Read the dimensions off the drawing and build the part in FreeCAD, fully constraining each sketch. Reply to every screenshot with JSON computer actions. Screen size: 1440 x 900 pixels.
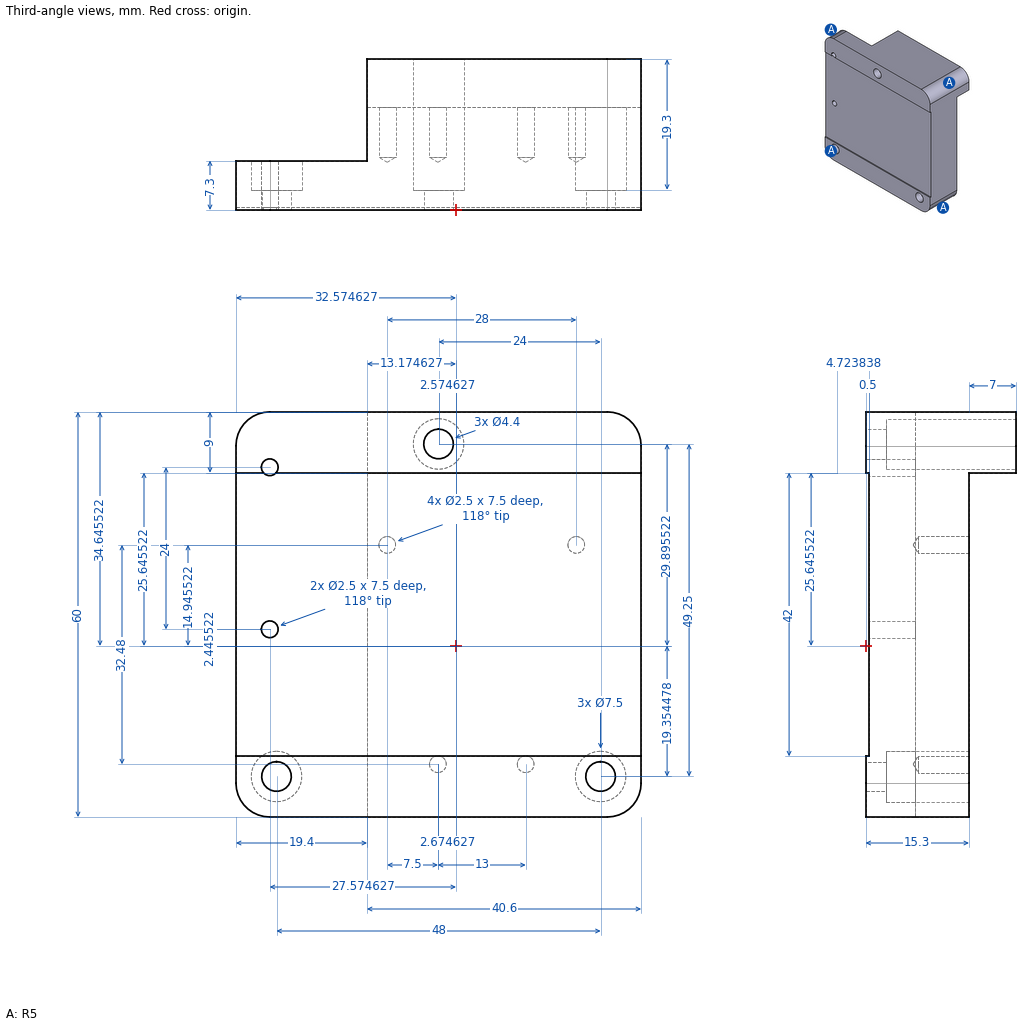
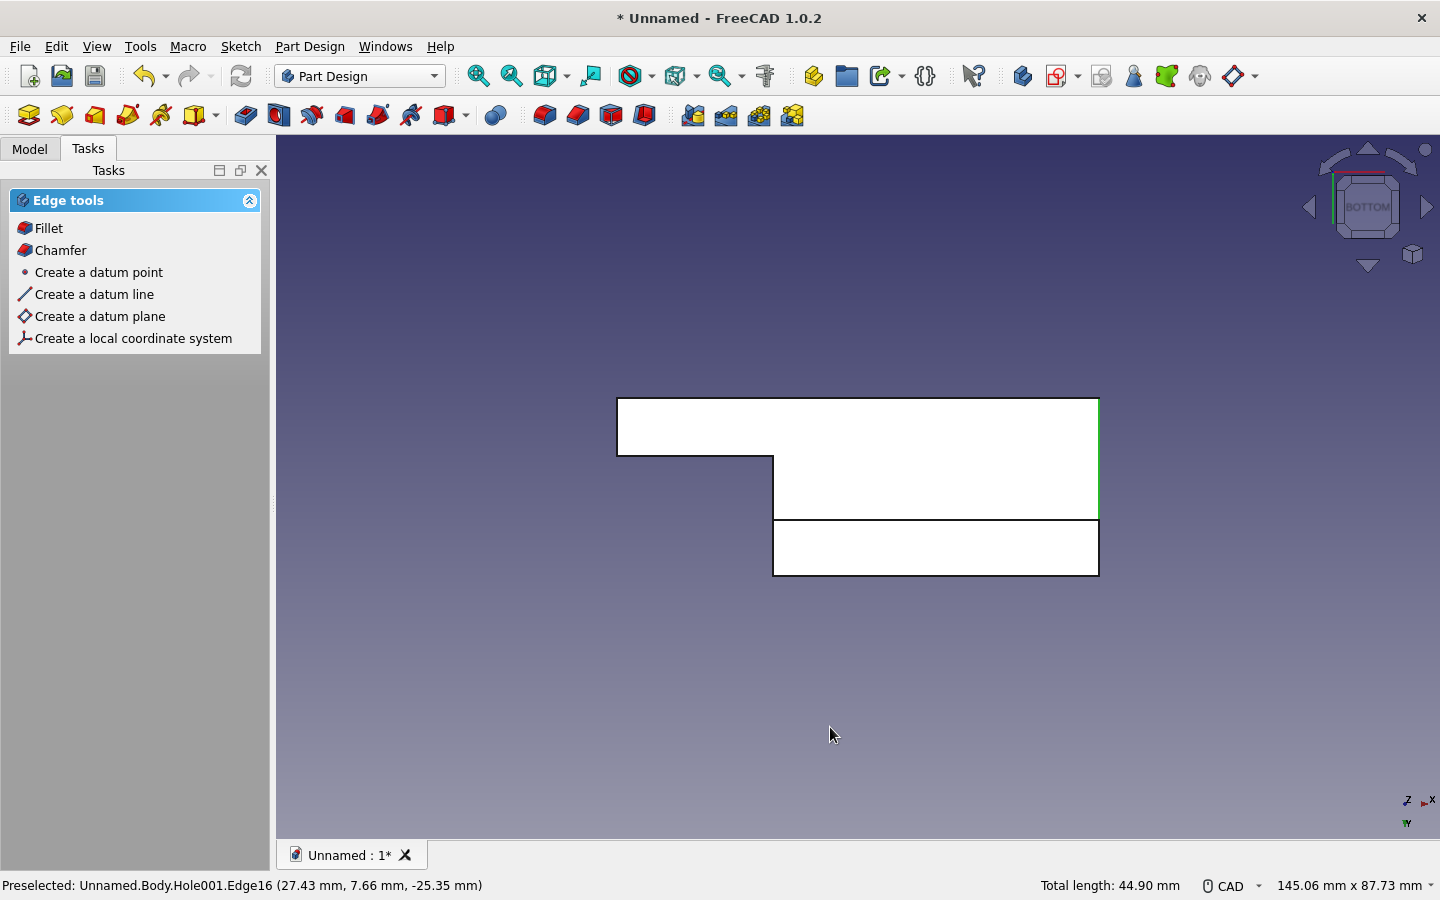
{"action": "key", "text": "v f"}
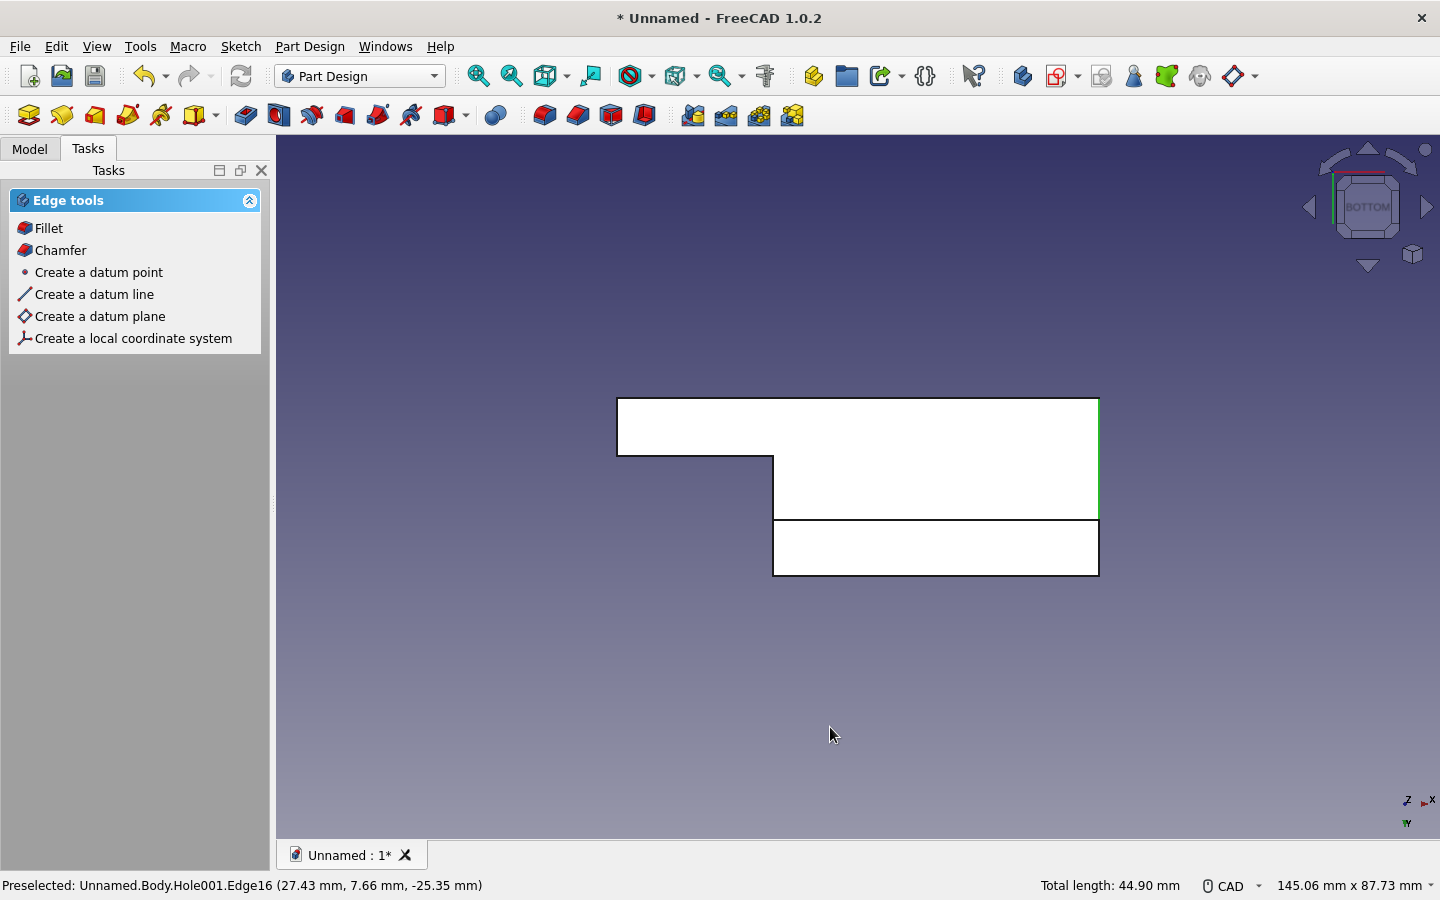
{"action": "left_click", "coordinate": [617, 426], "text": "ctrl"}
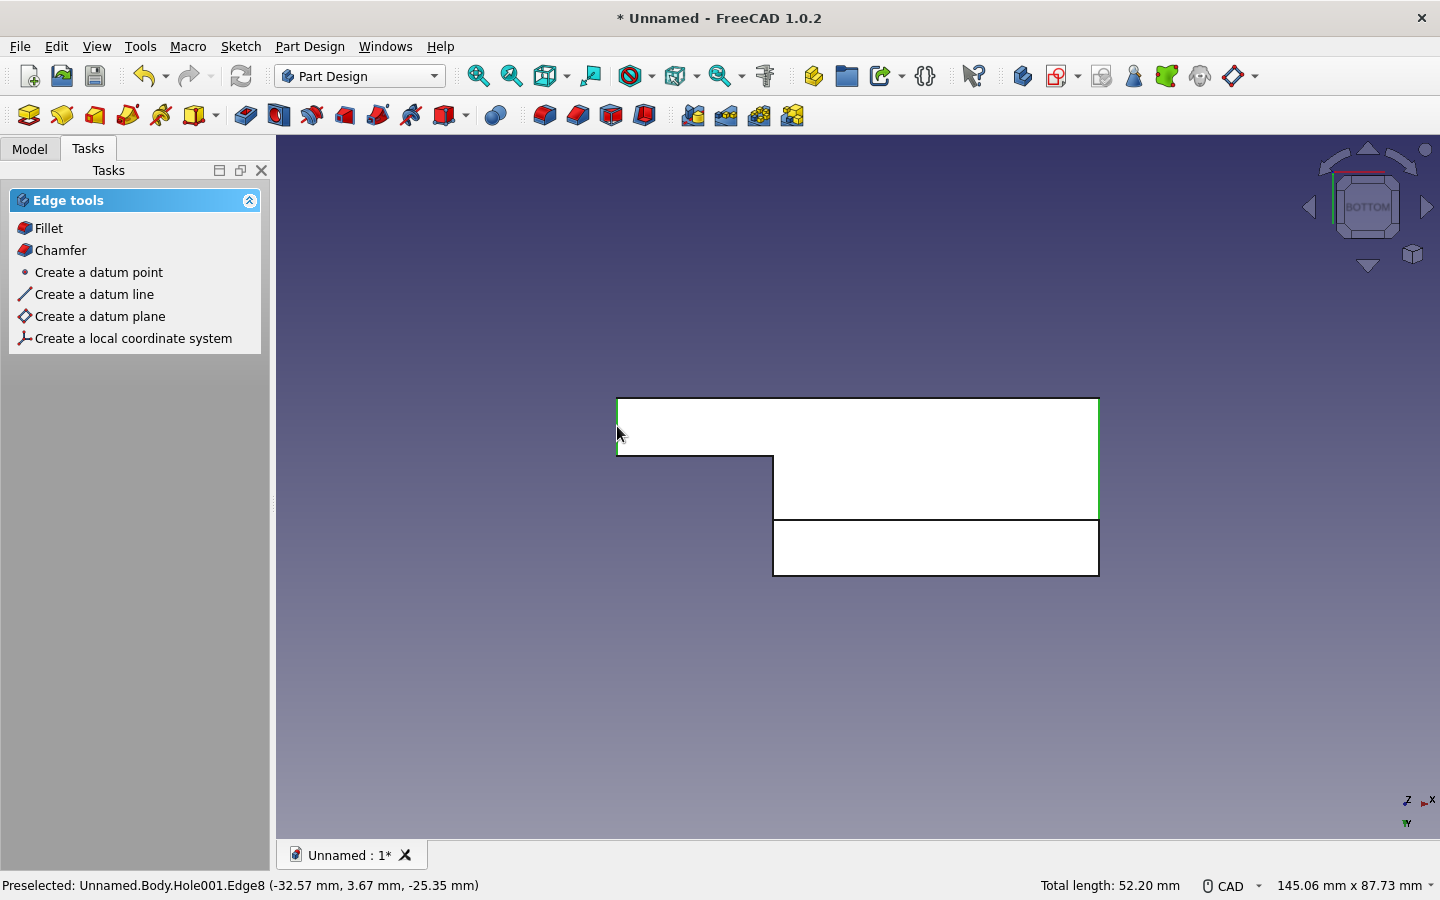
{"action": "left_click", "coordinate": [545, 116]}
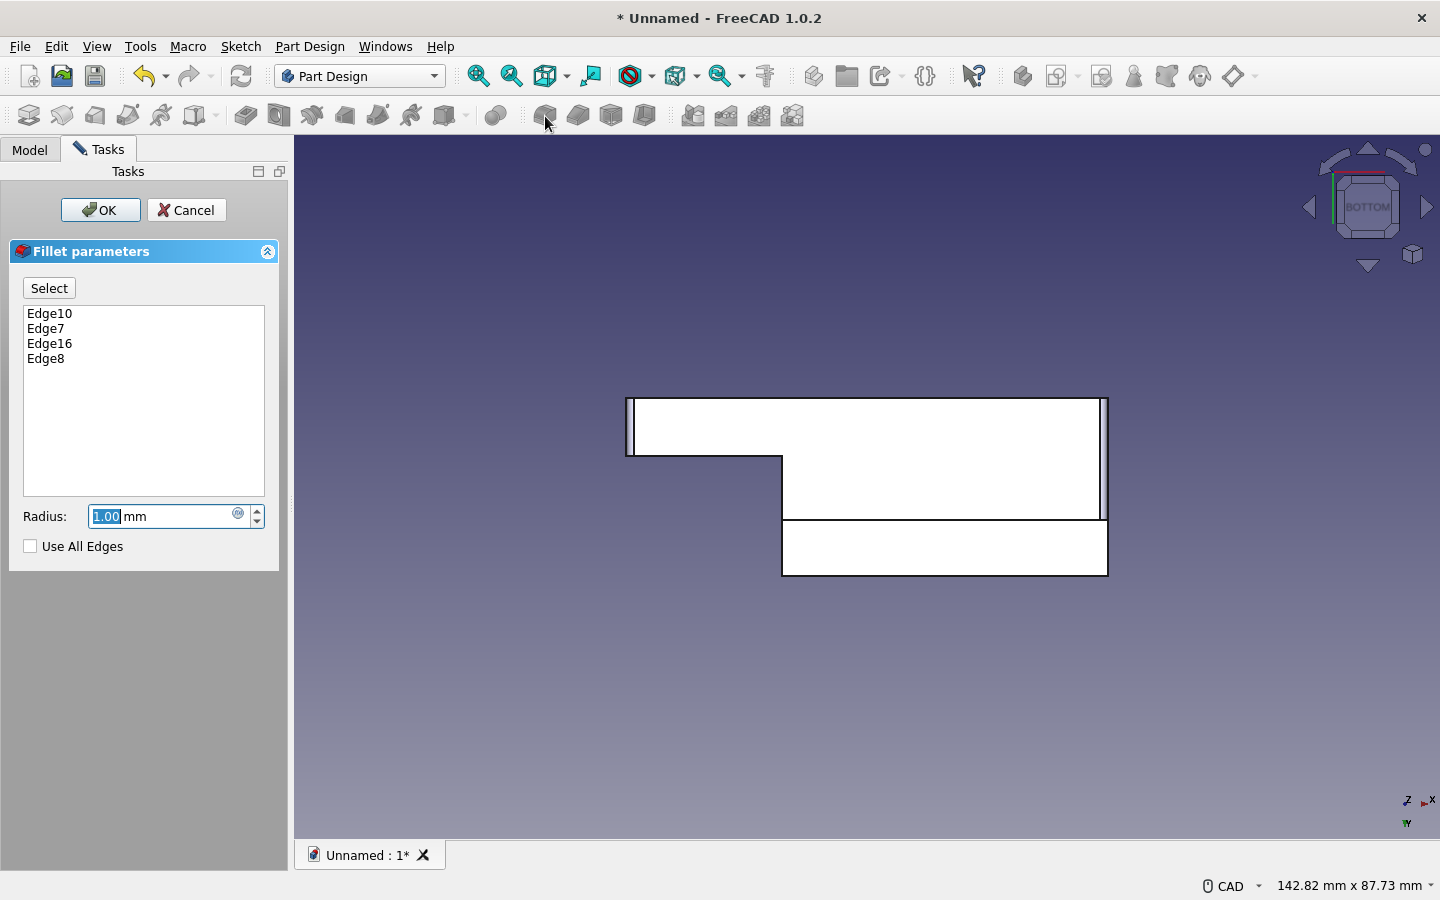
{"action": "type", "text": "5"}
{"action": "key", "text": "Tab"}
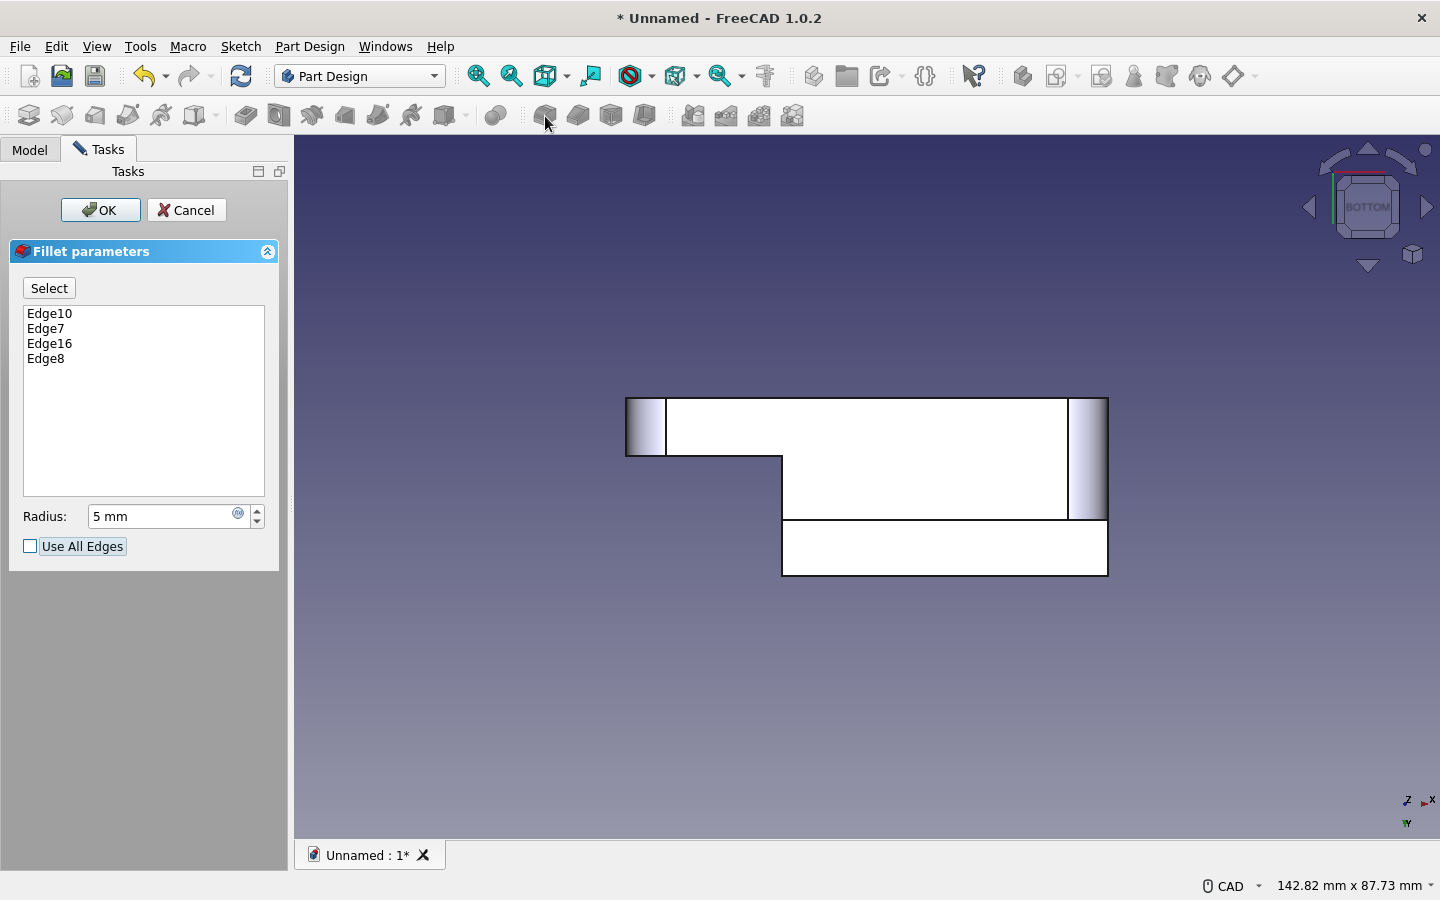
{"action": "left_click", "coordinate": [101, 210]}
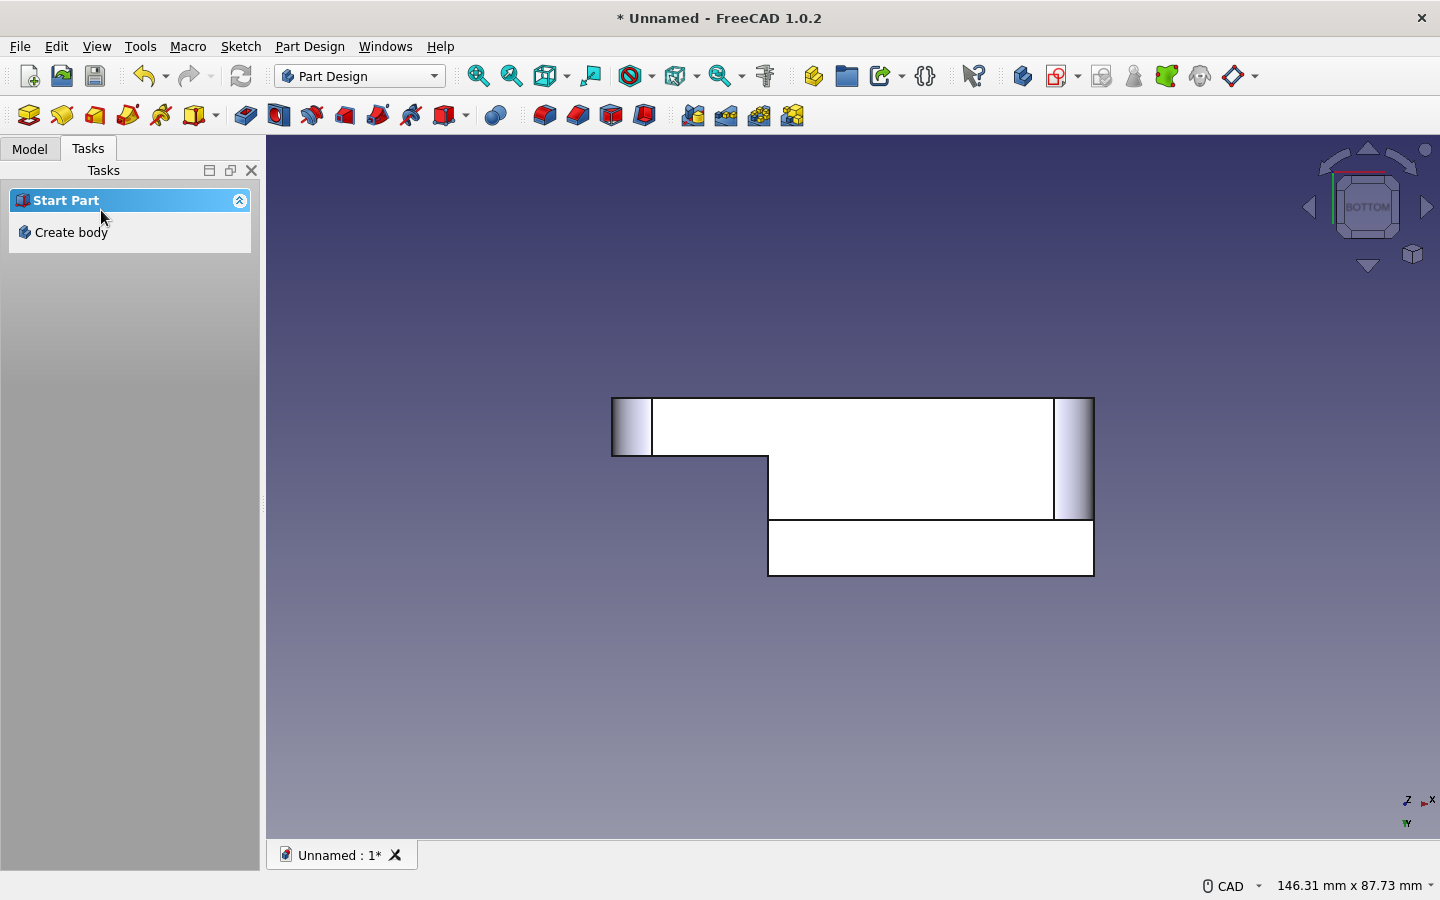
{"action": "left_click", "coordinate": [479, 76]}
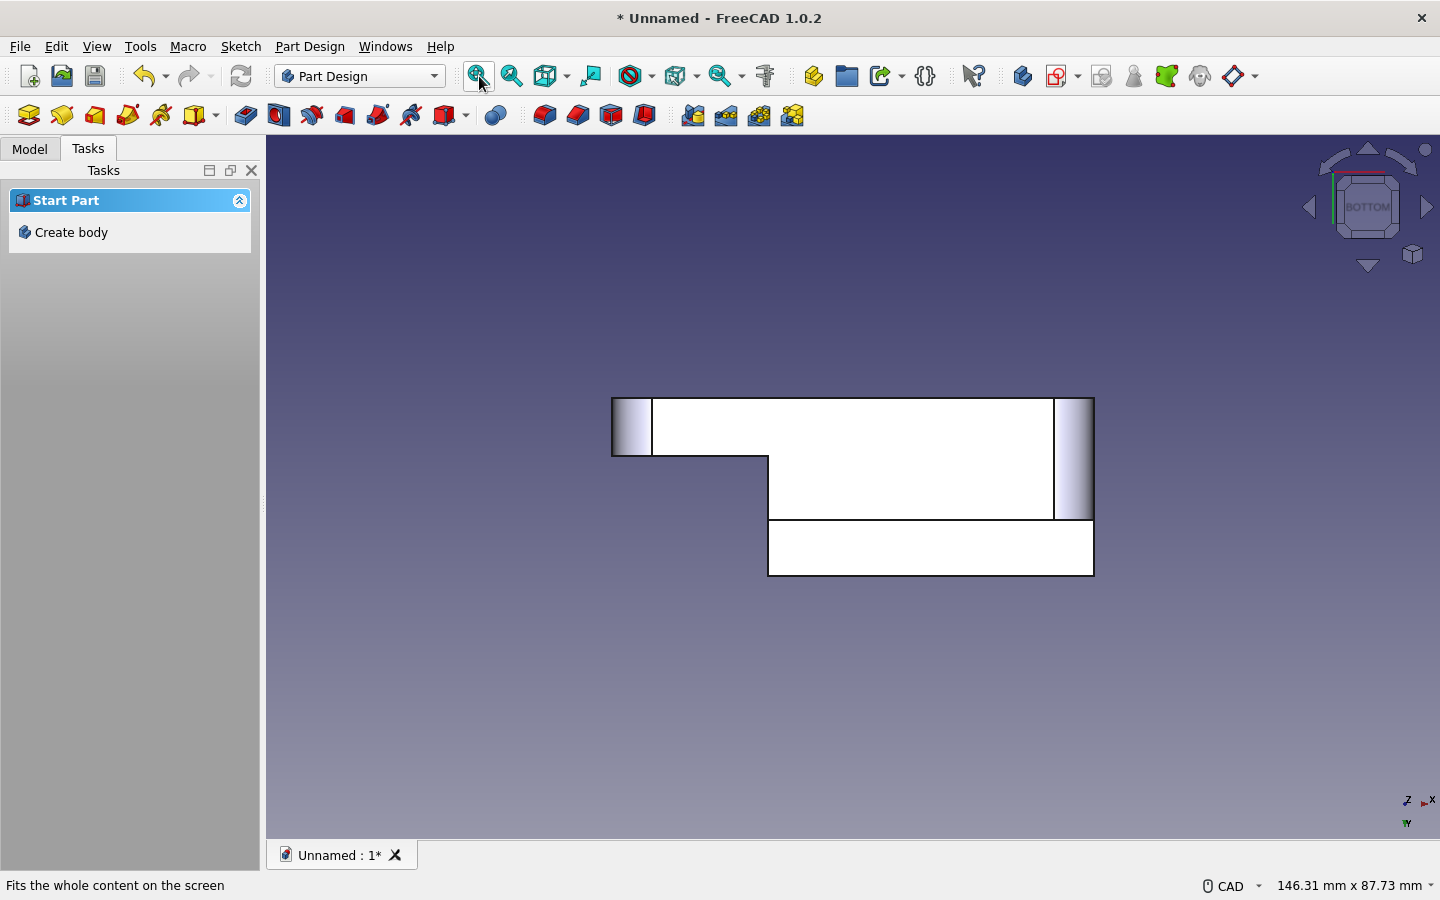
{"action": "key", "text": "6"}